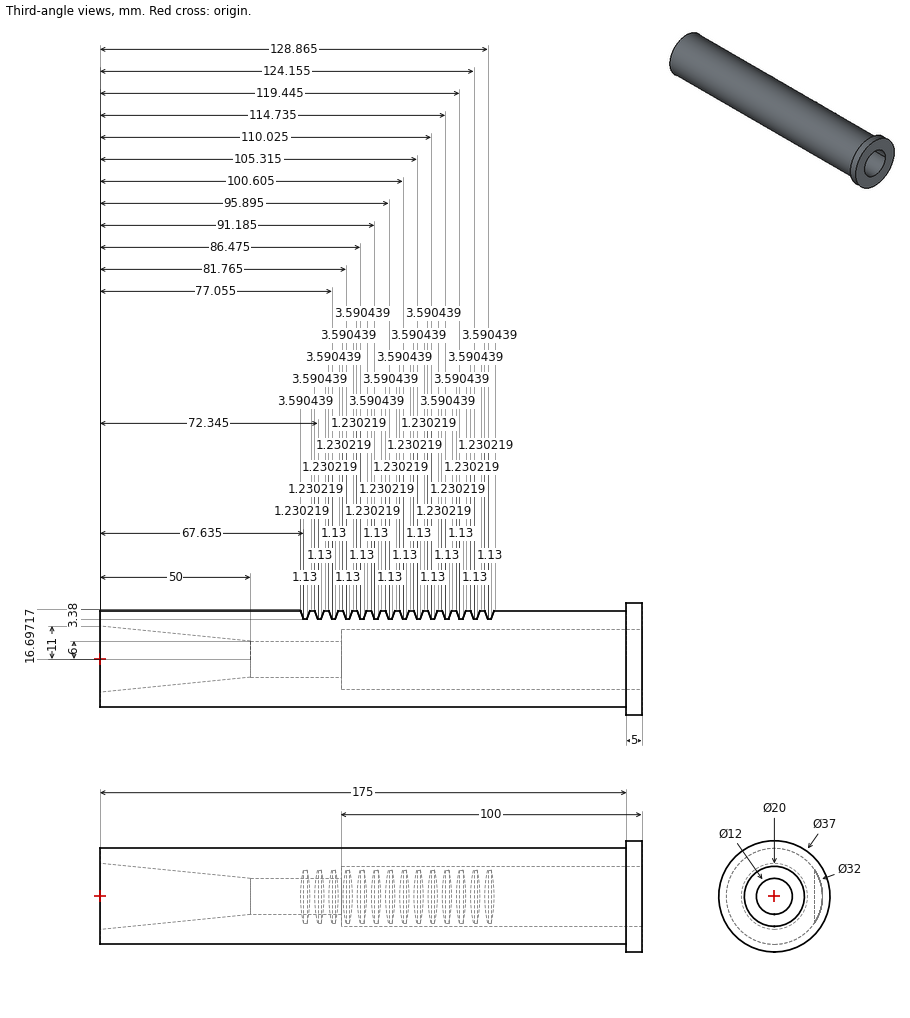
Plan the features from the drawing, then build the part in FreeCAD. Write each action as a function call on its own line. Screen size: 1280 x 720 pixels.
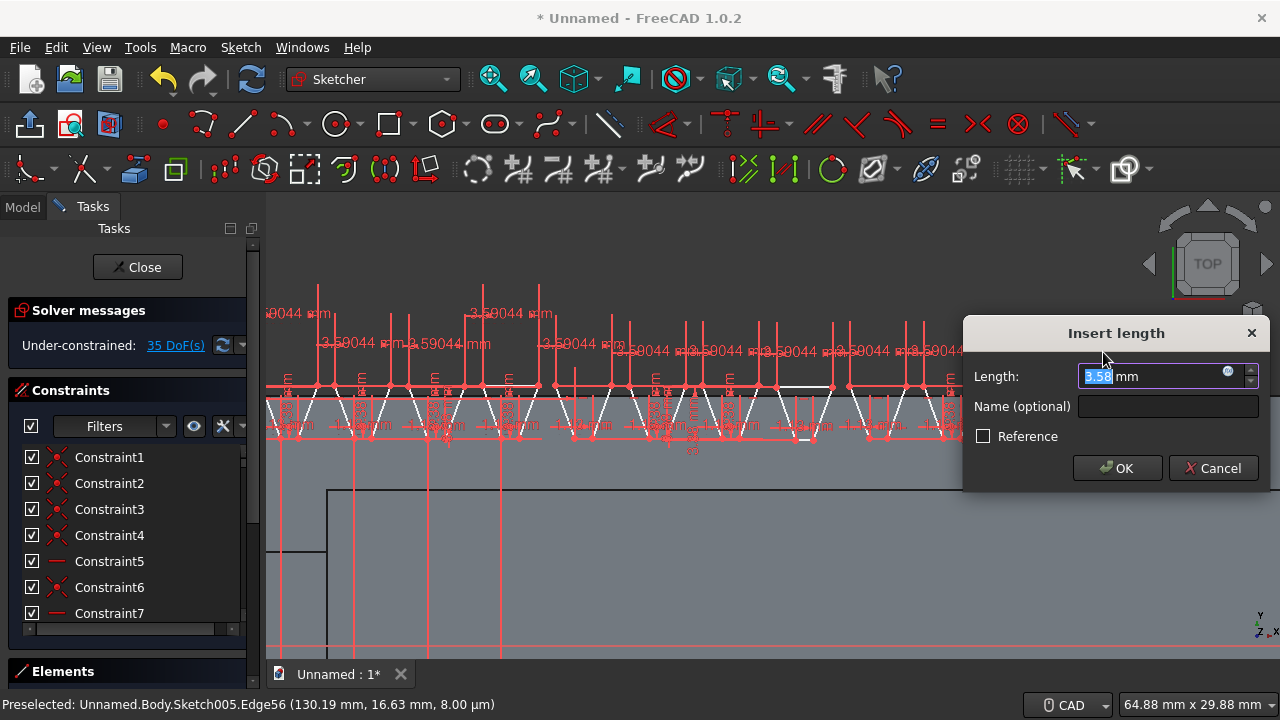
text(3.590439)
key(Return)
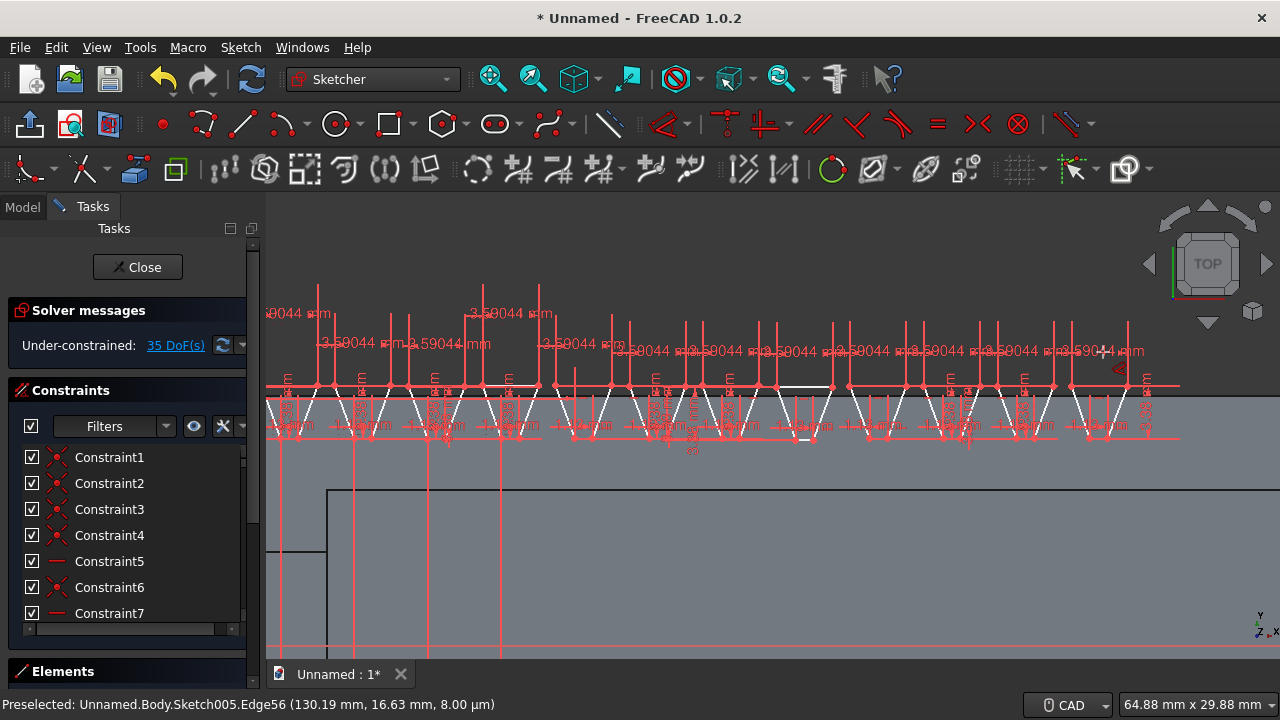
click(649, 439)
click(390, 309)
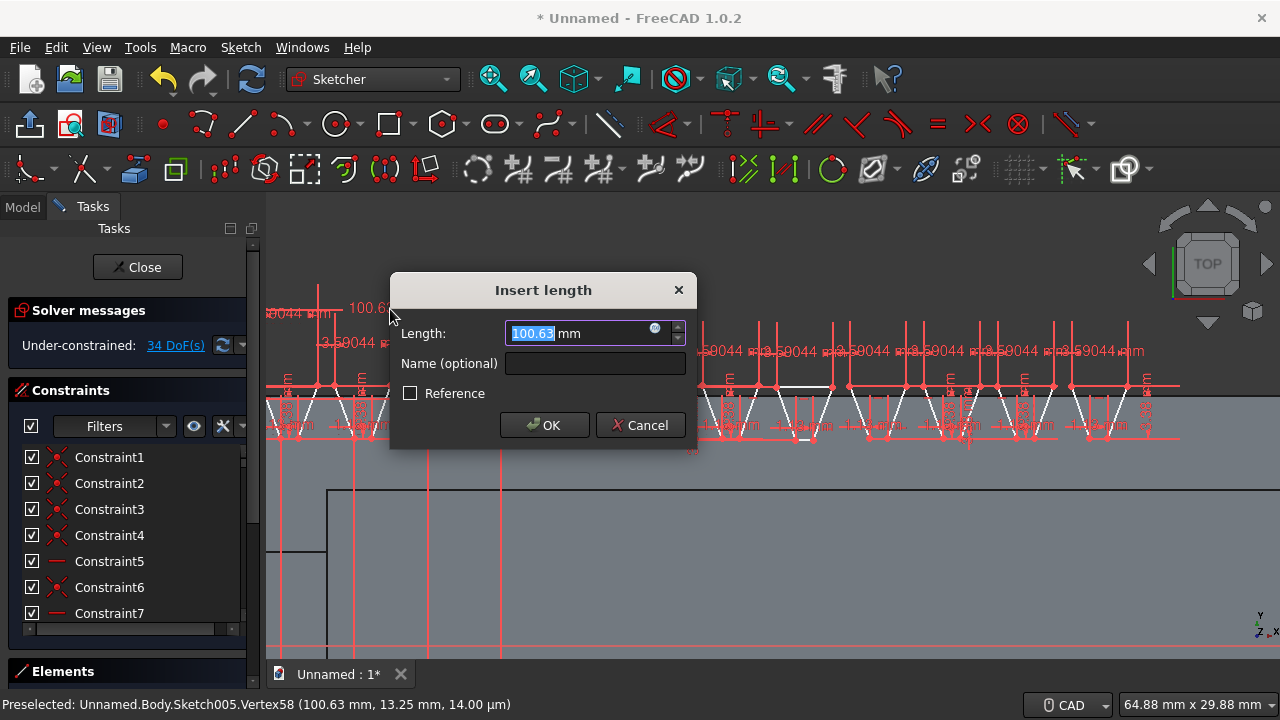
text(100.605)
key(Return)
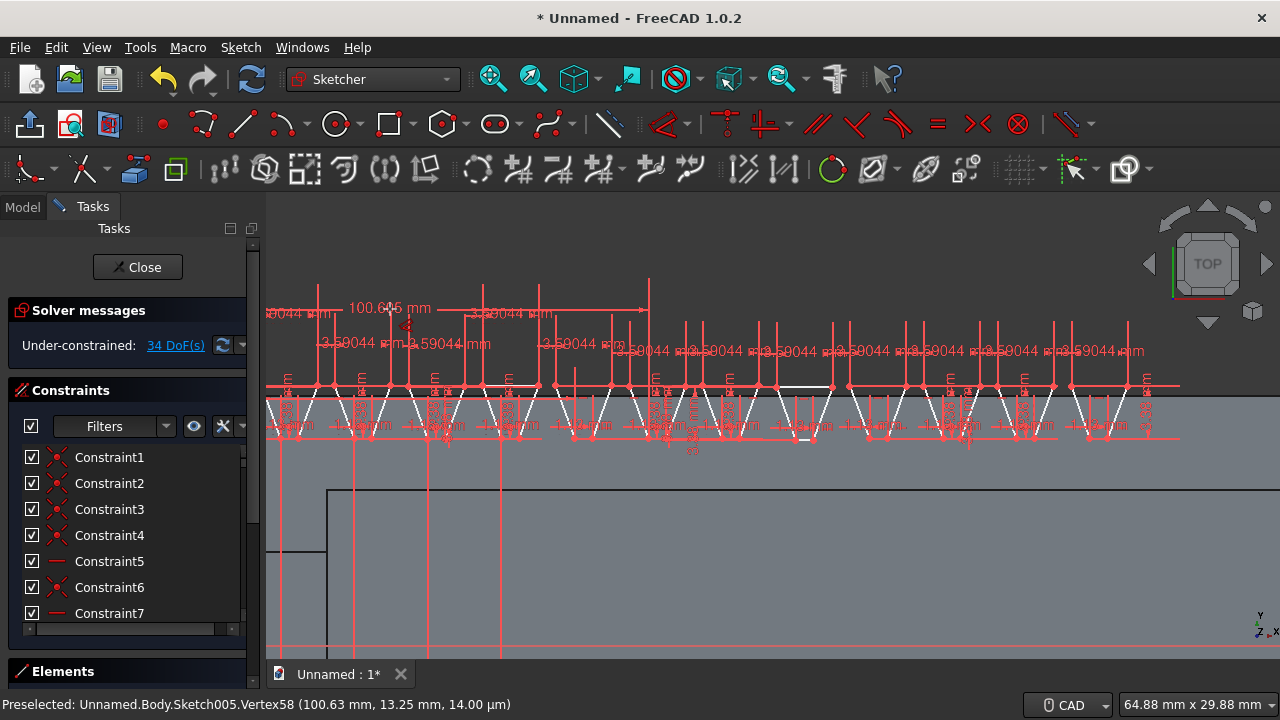
click(722, 439)
click(606, 309)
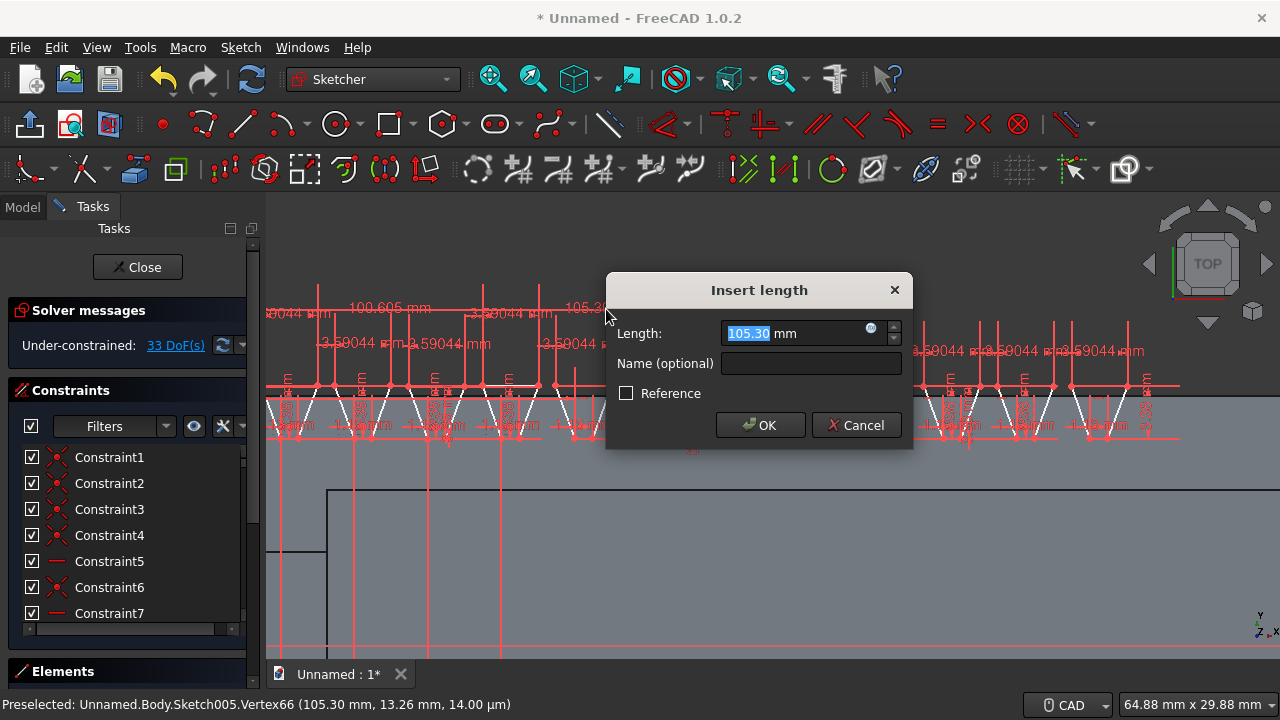
text(105.315)
key(Return)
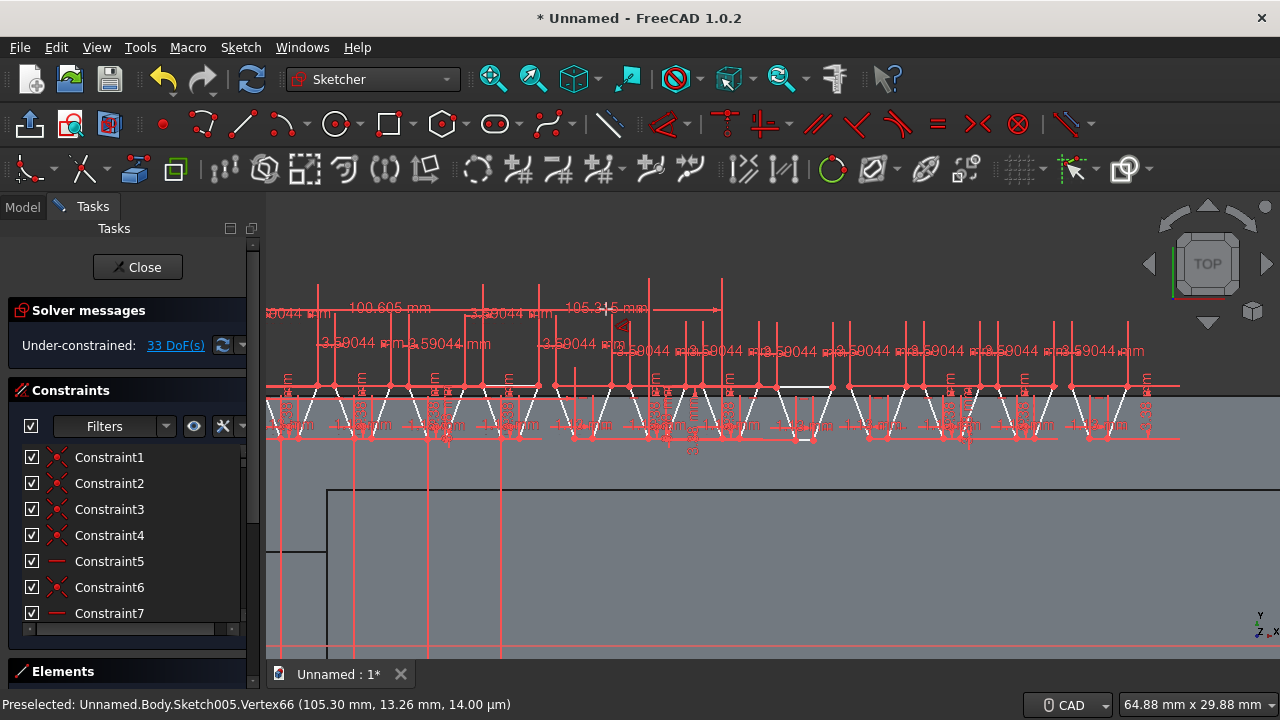
click(796, 440)
click(720, 310)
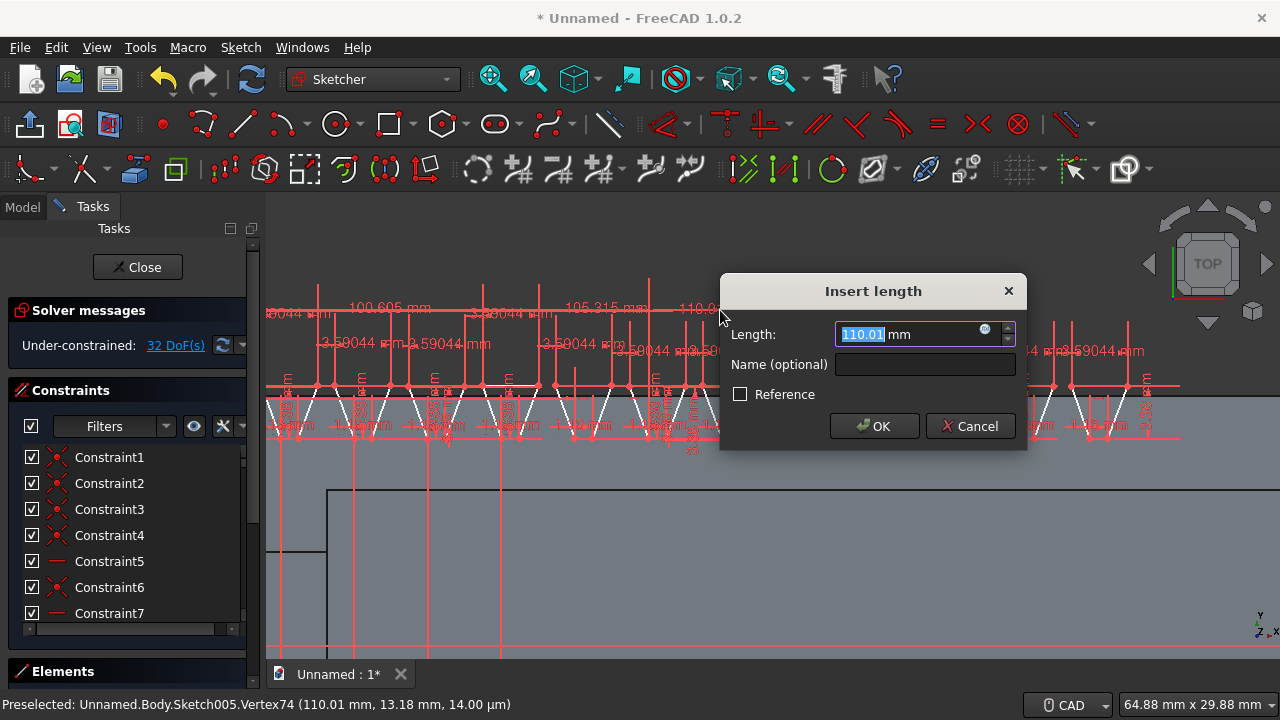
text(110.025)
key(Return)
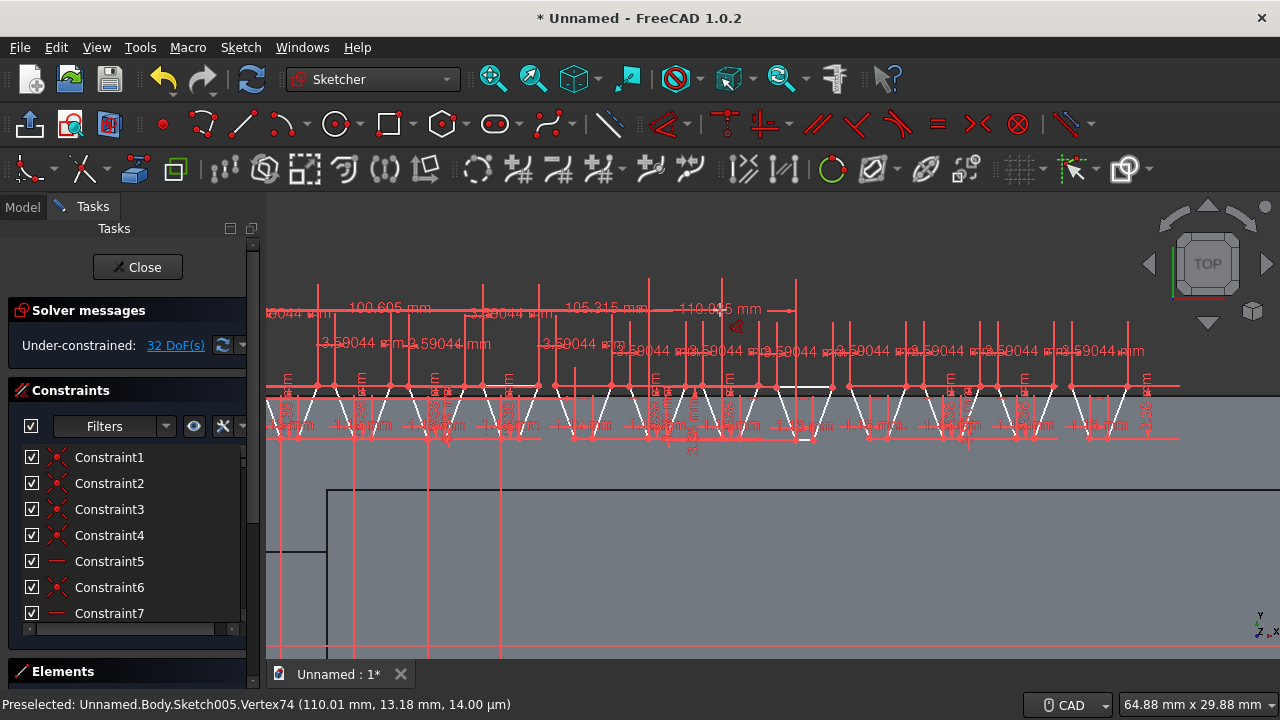
click(870, 439)
click(582, 405)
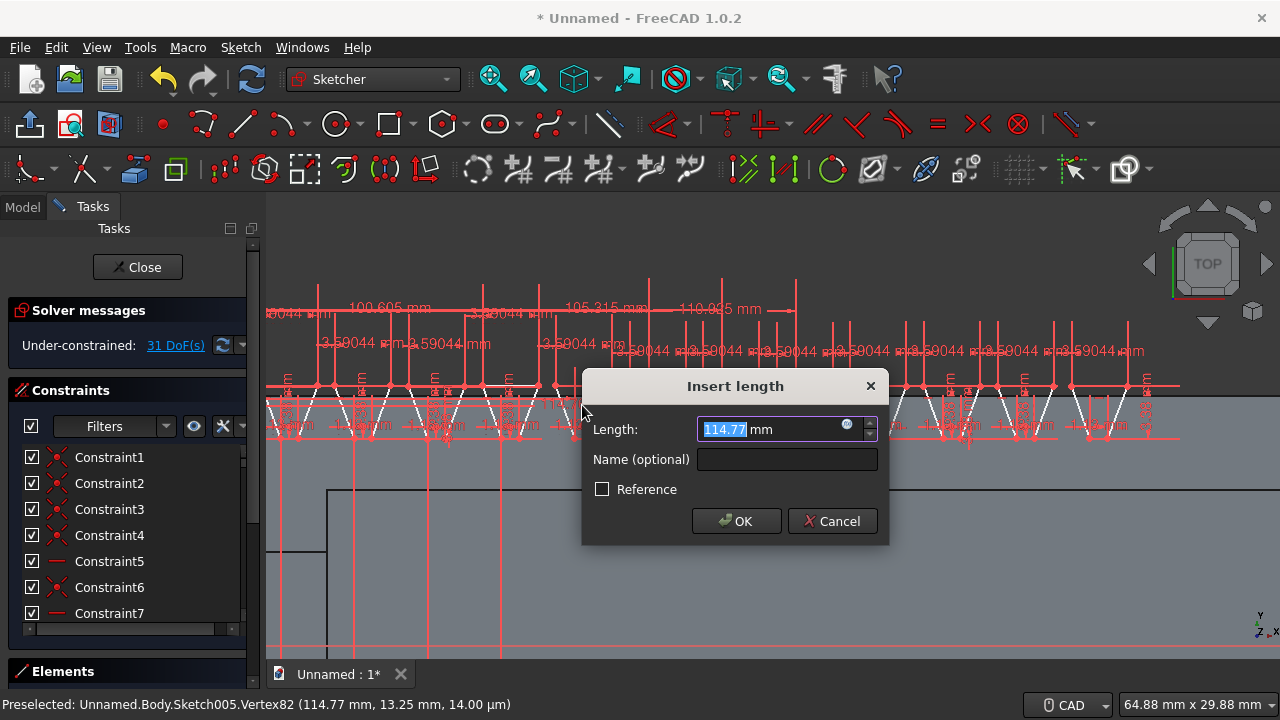
text(114.735)
key(Return)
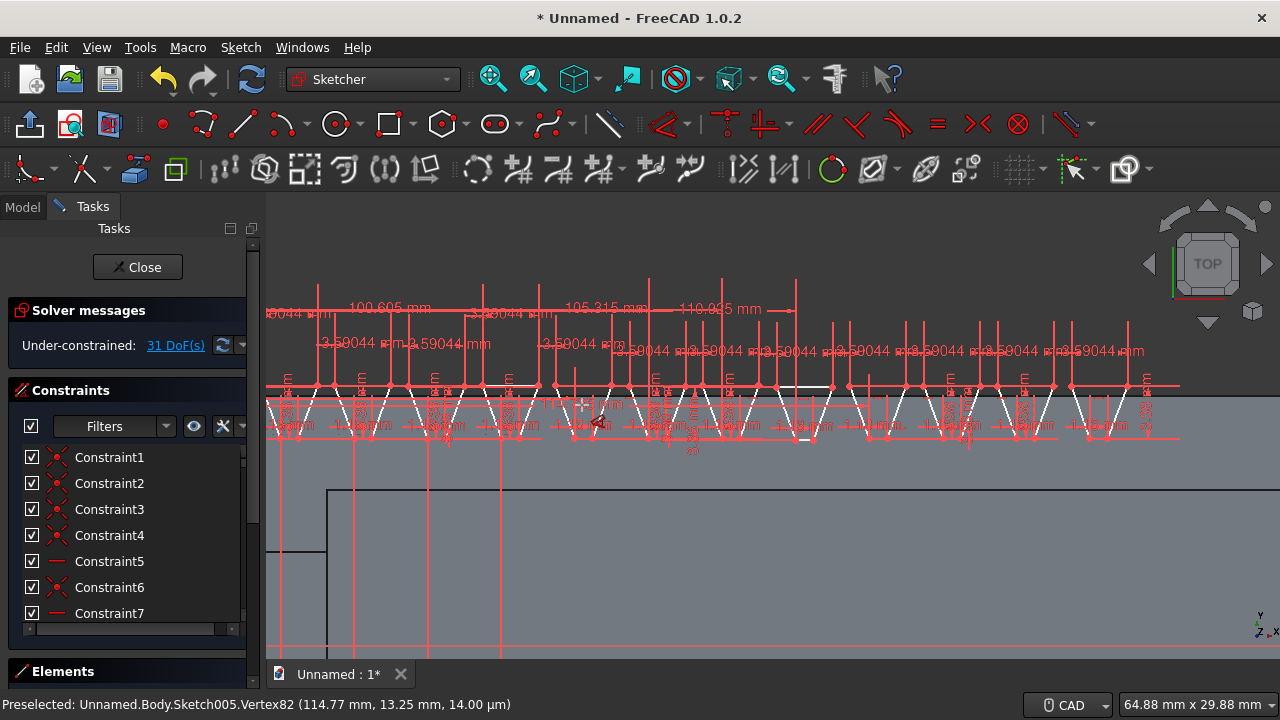
click(943, 439)
click(846, 309)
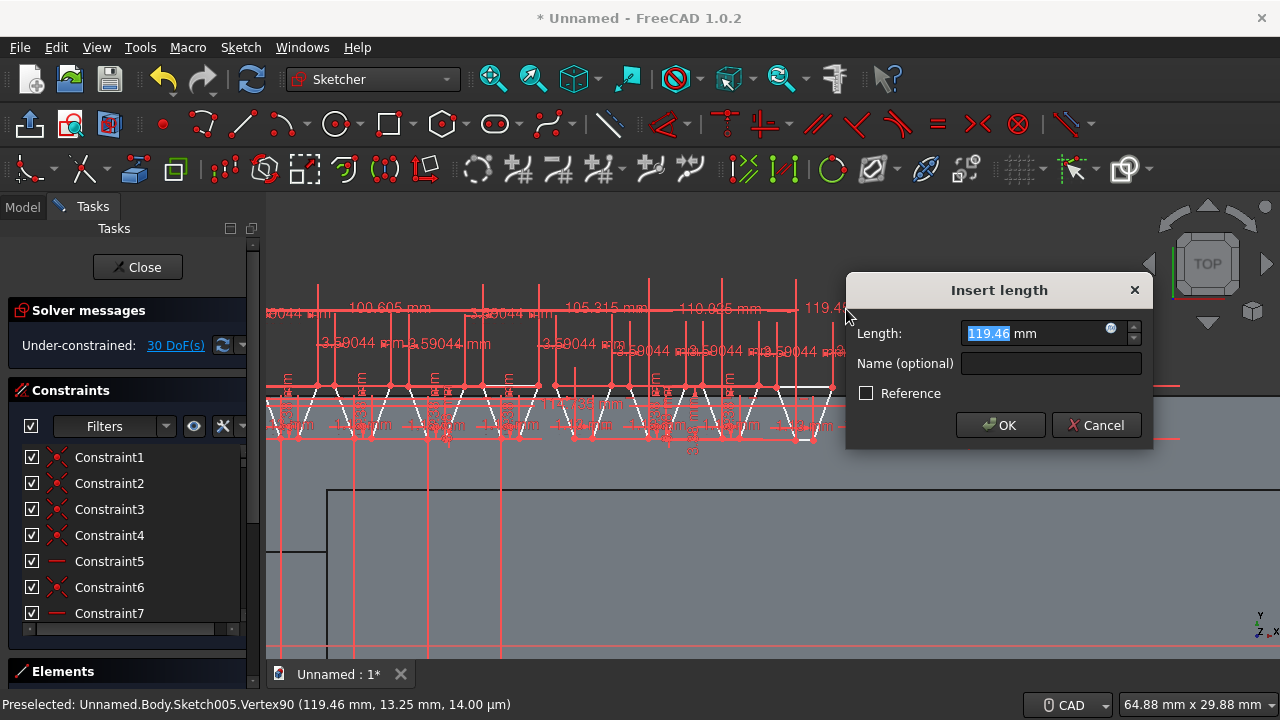
text(119.445)
key(Return)